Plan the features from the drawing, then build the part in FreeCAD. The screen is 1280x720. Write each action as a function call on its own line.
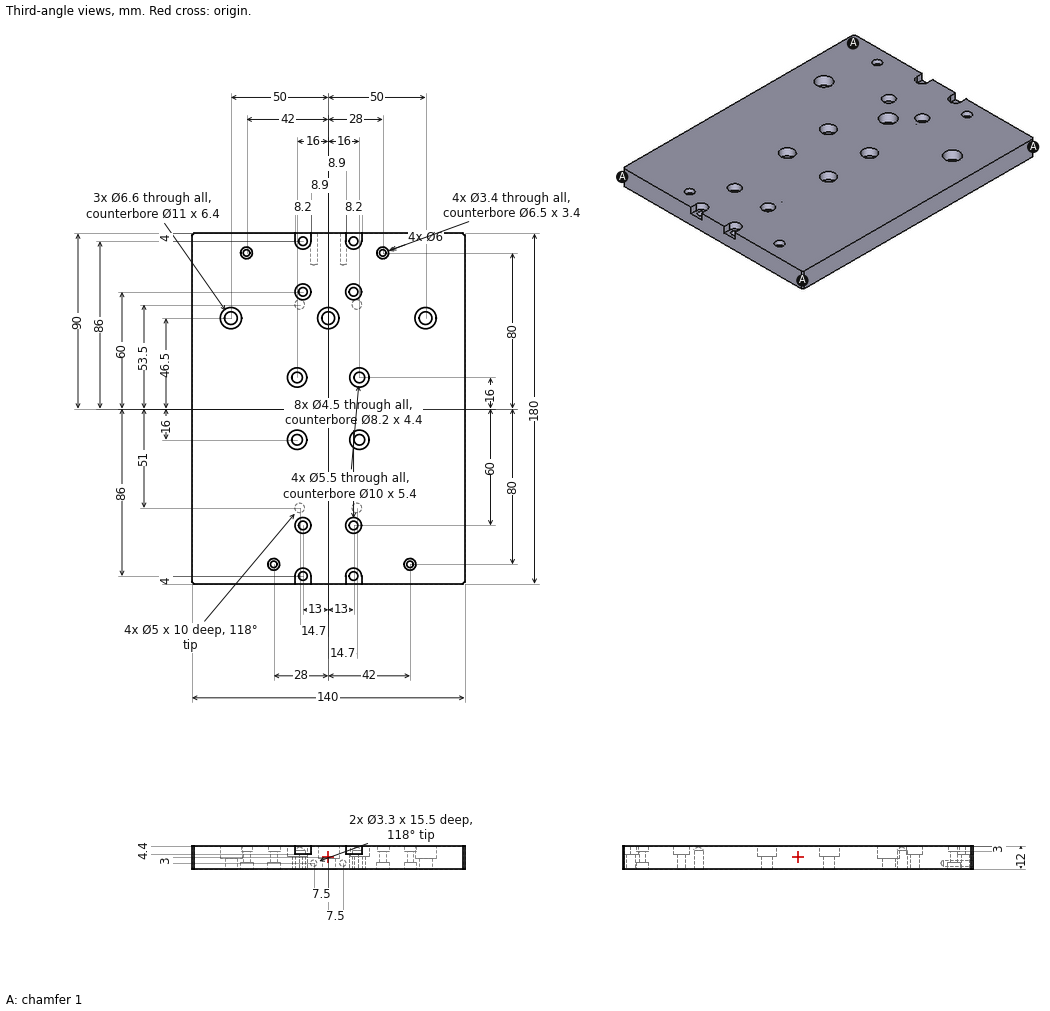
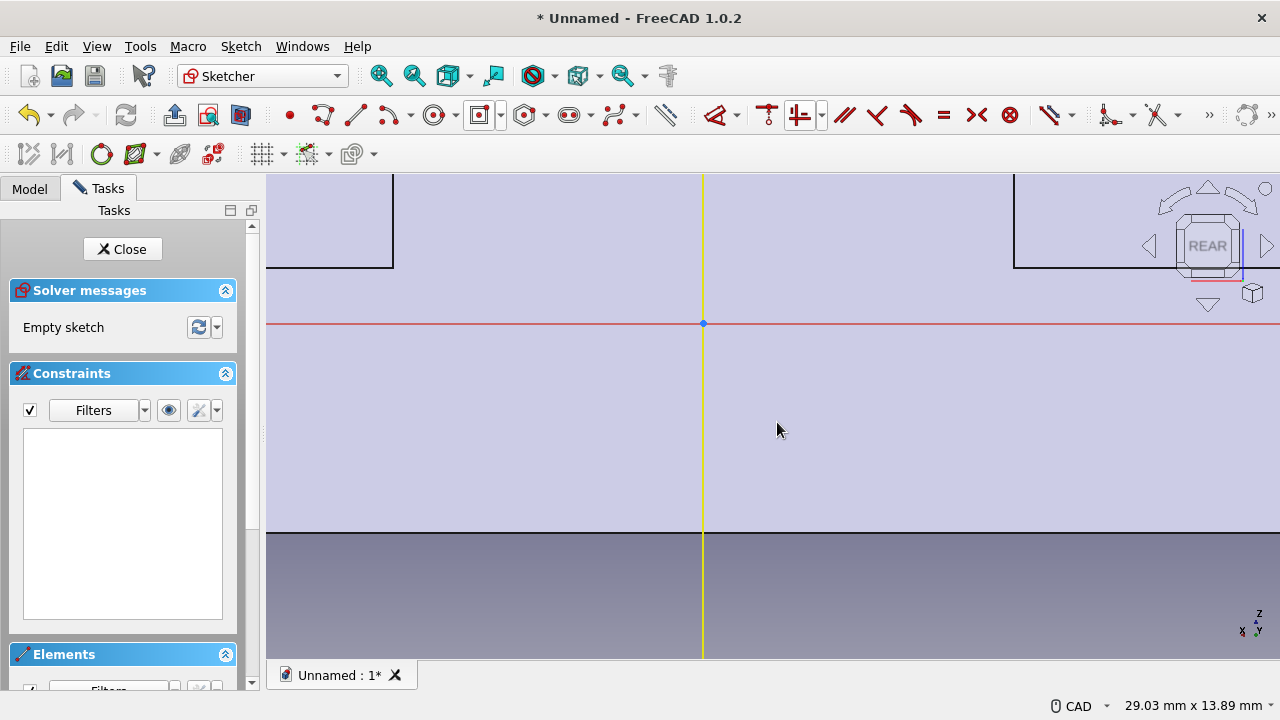
click(434, 116)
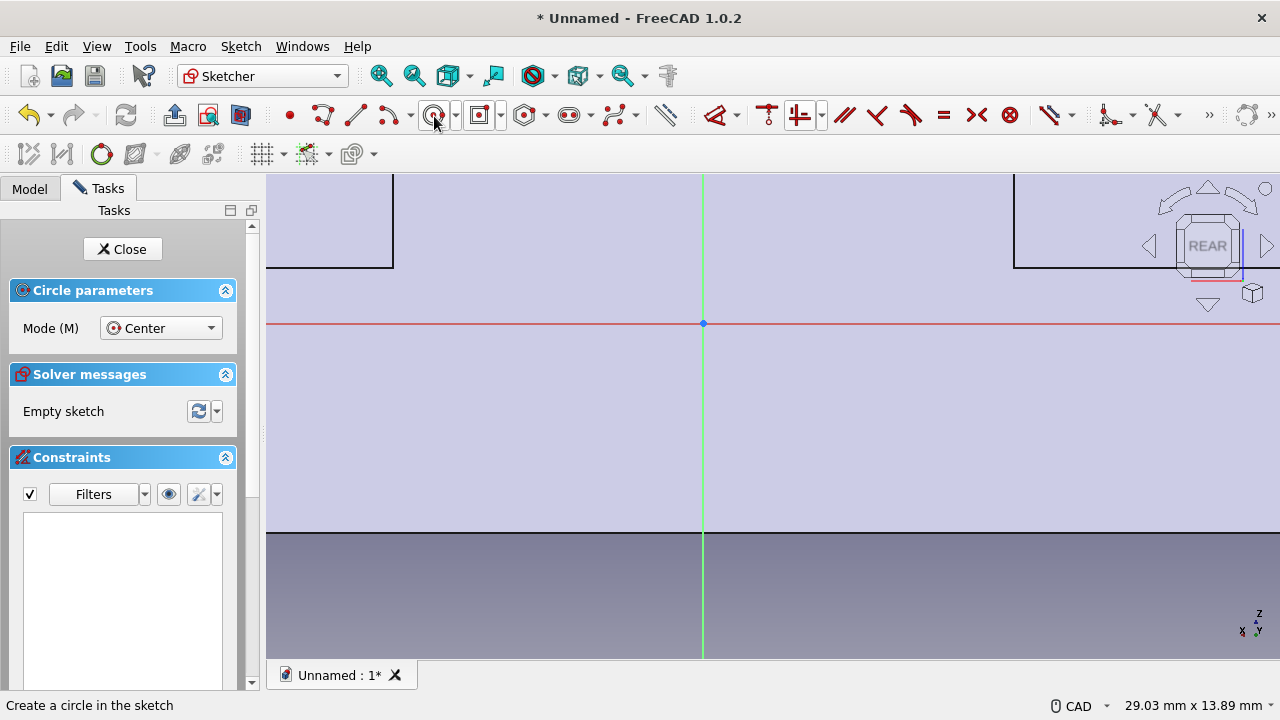
click(965, 428)
click(1006, 388)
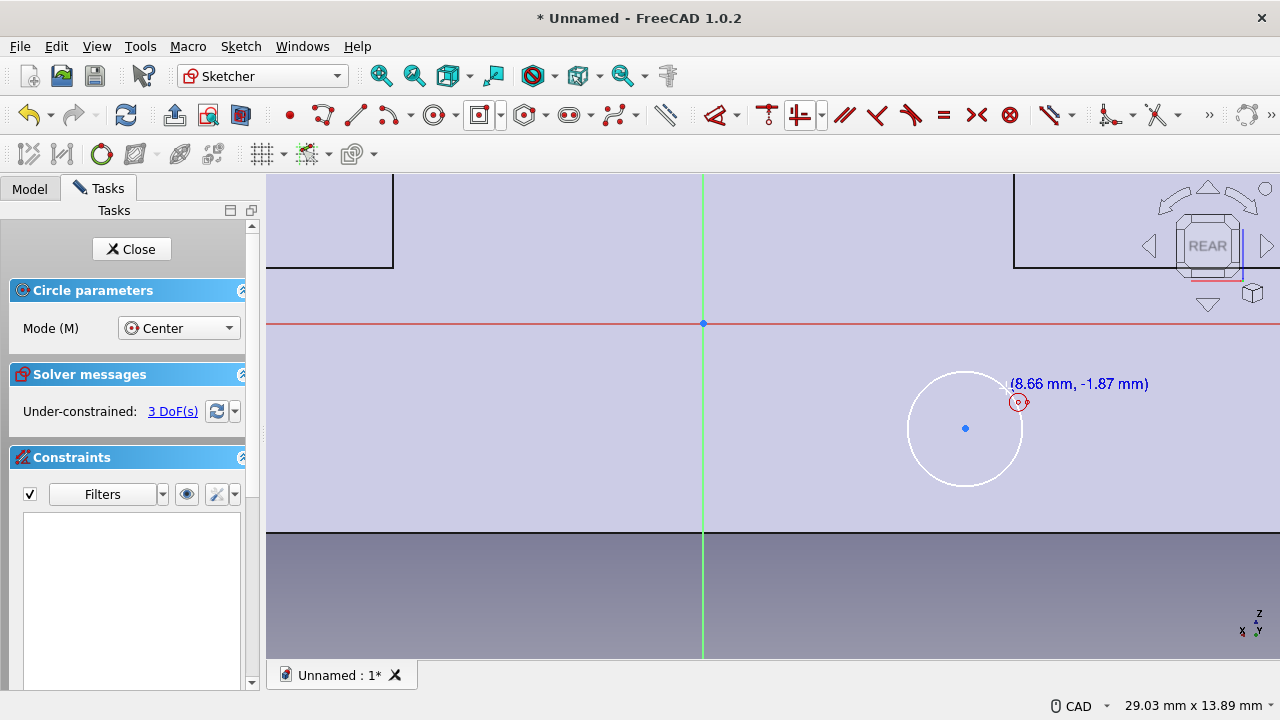
click(441, 428)
click(482, 388)
key(Escape)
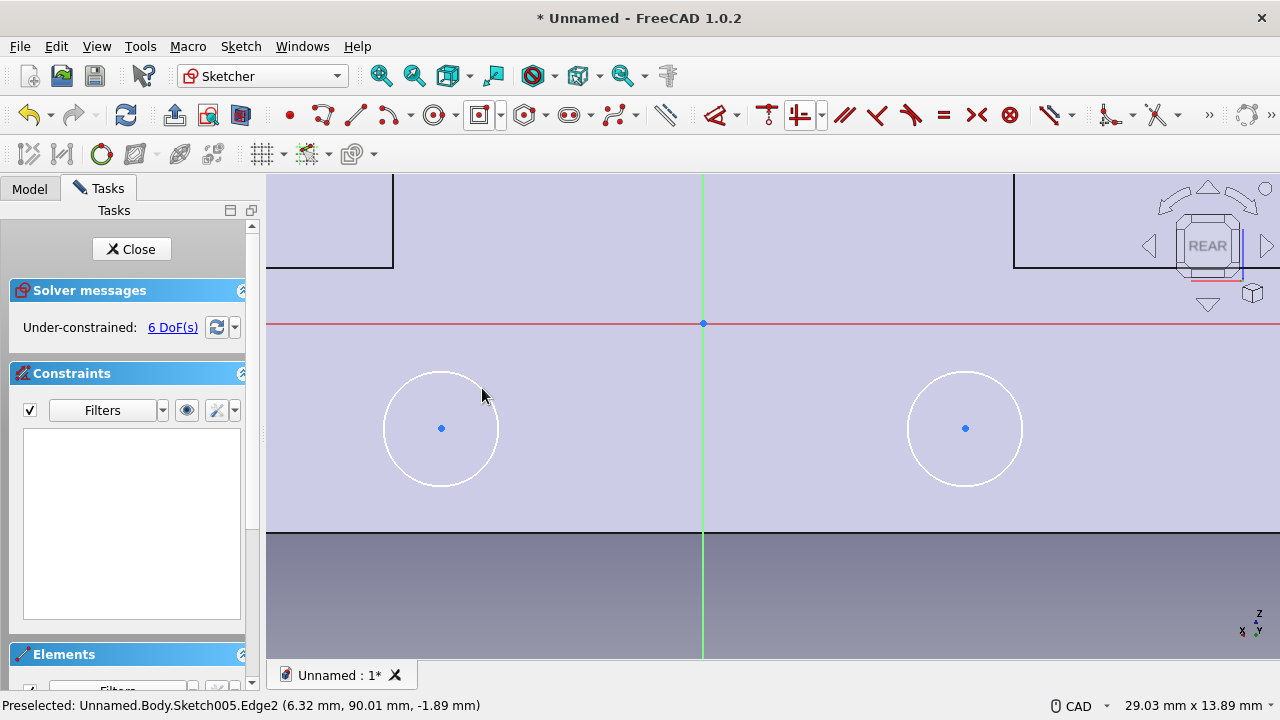
click(1005, 388)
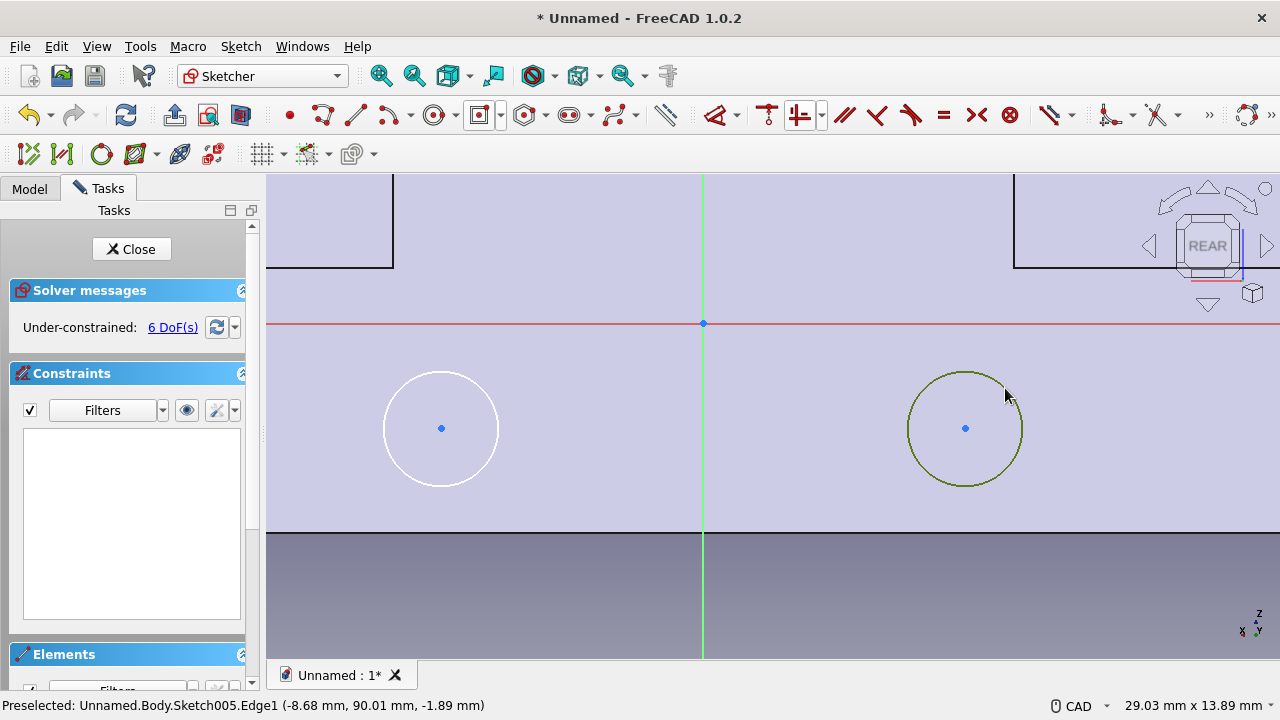
click(481, 388)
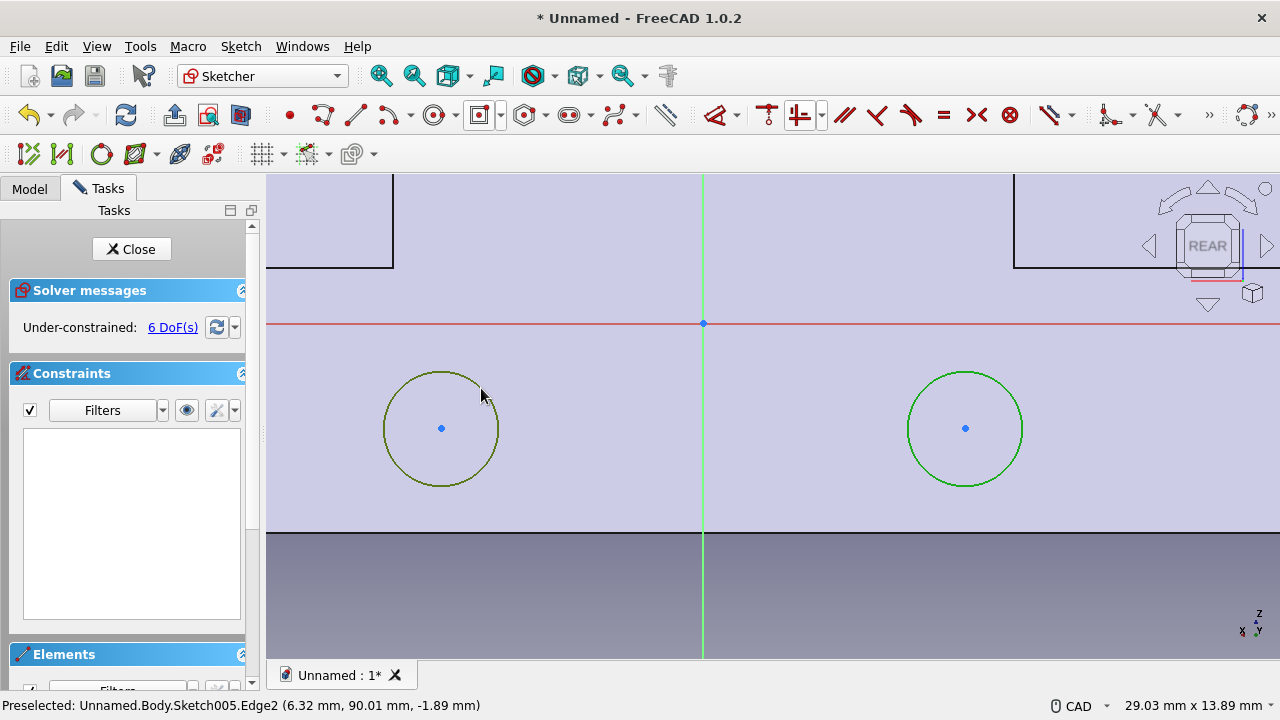
click(944, 116)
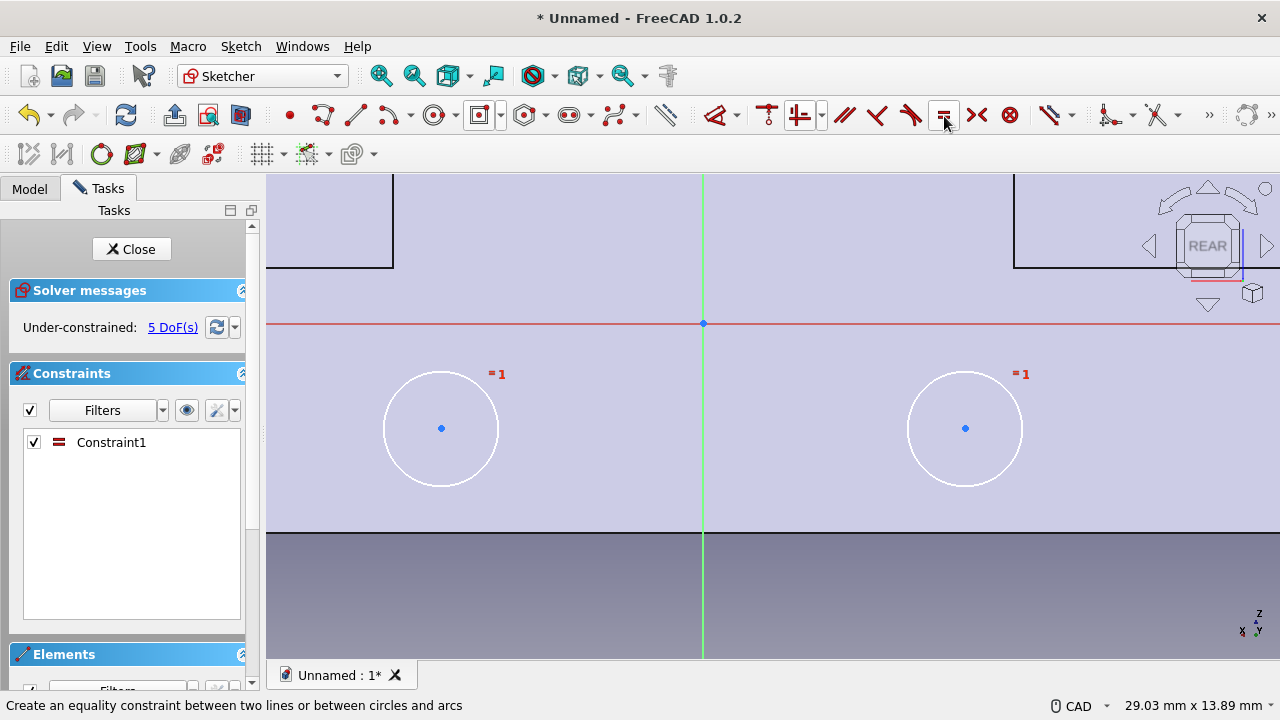
click(714, 116)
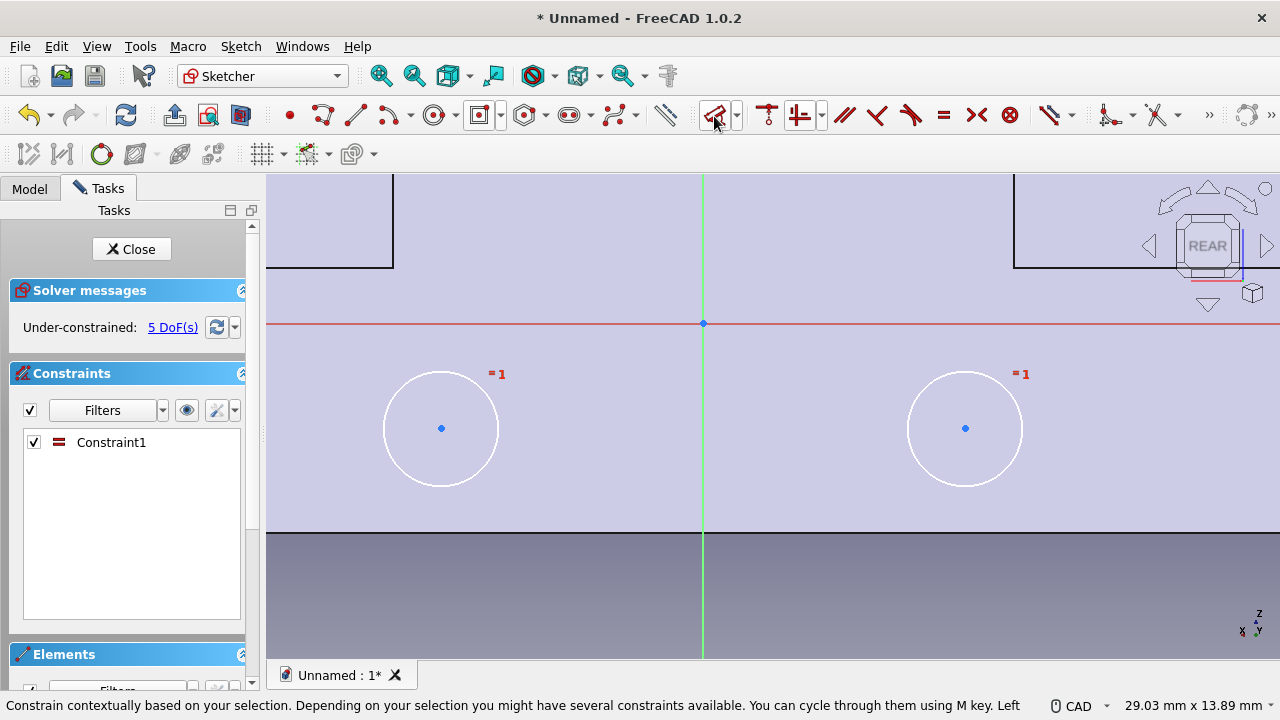
click(1005, 388)
click(1027, 365)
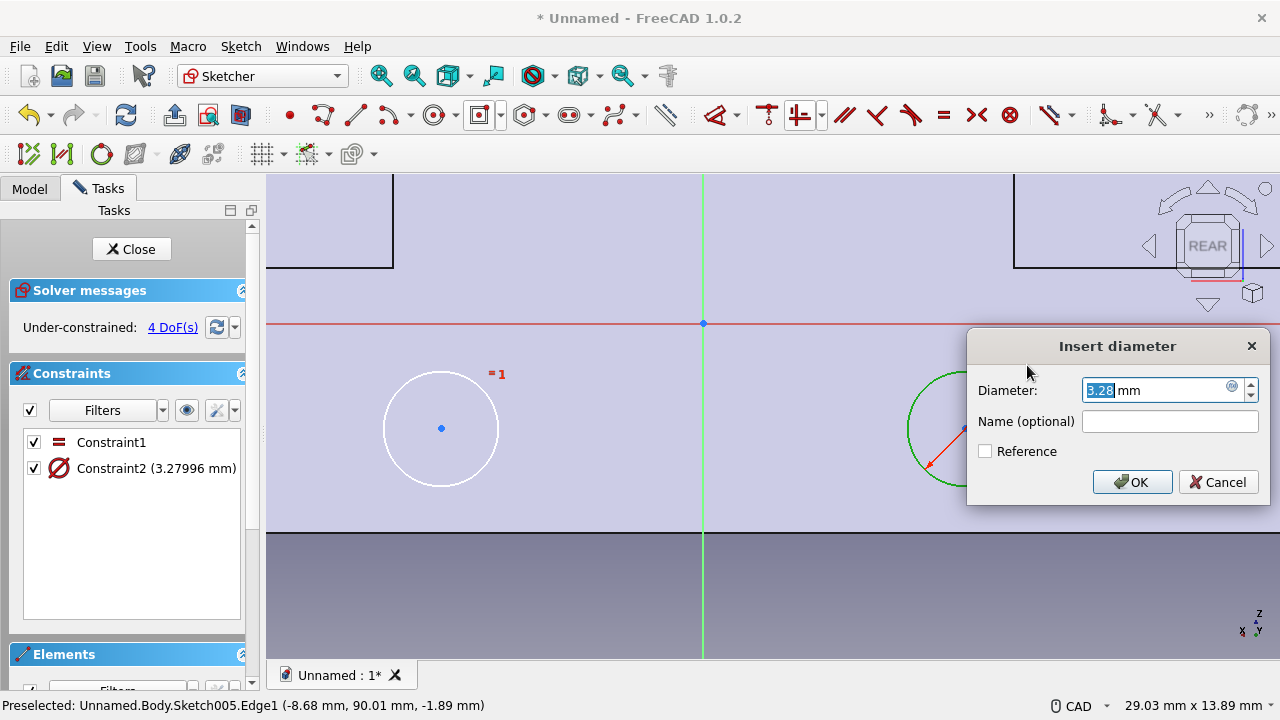
text(3.3)
key(Return)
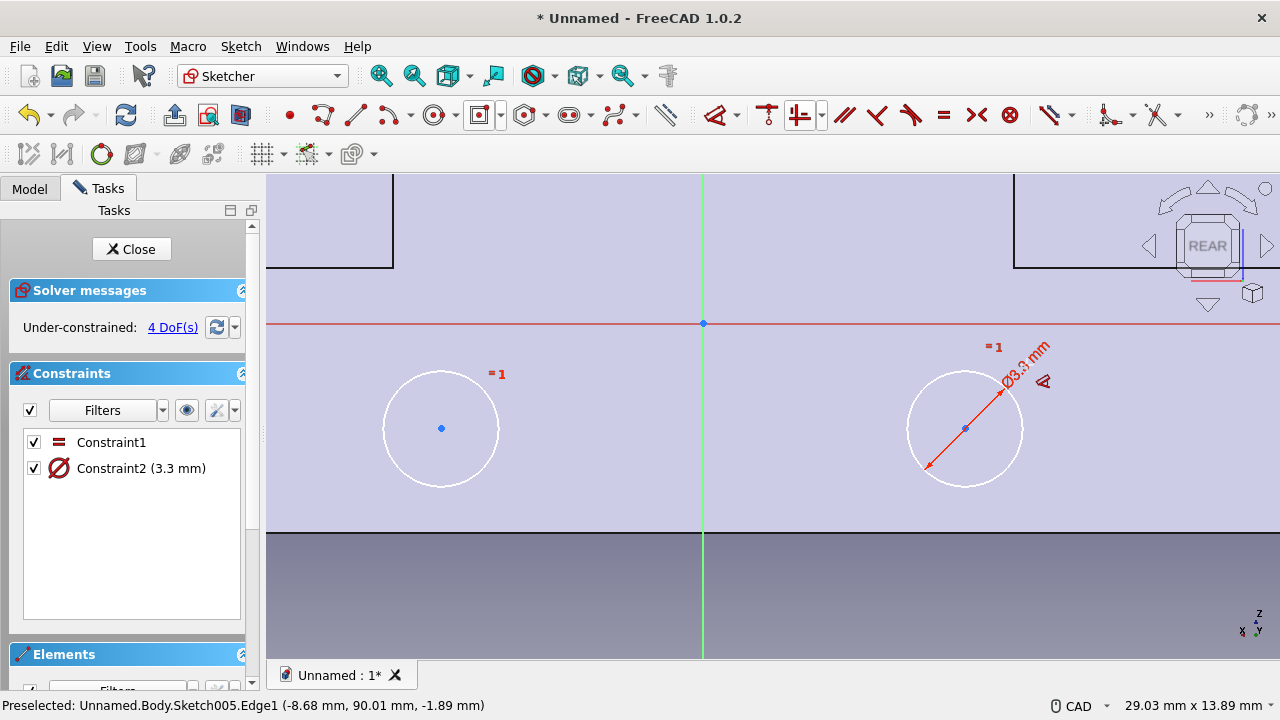
click(965, 429)
click(999, 401)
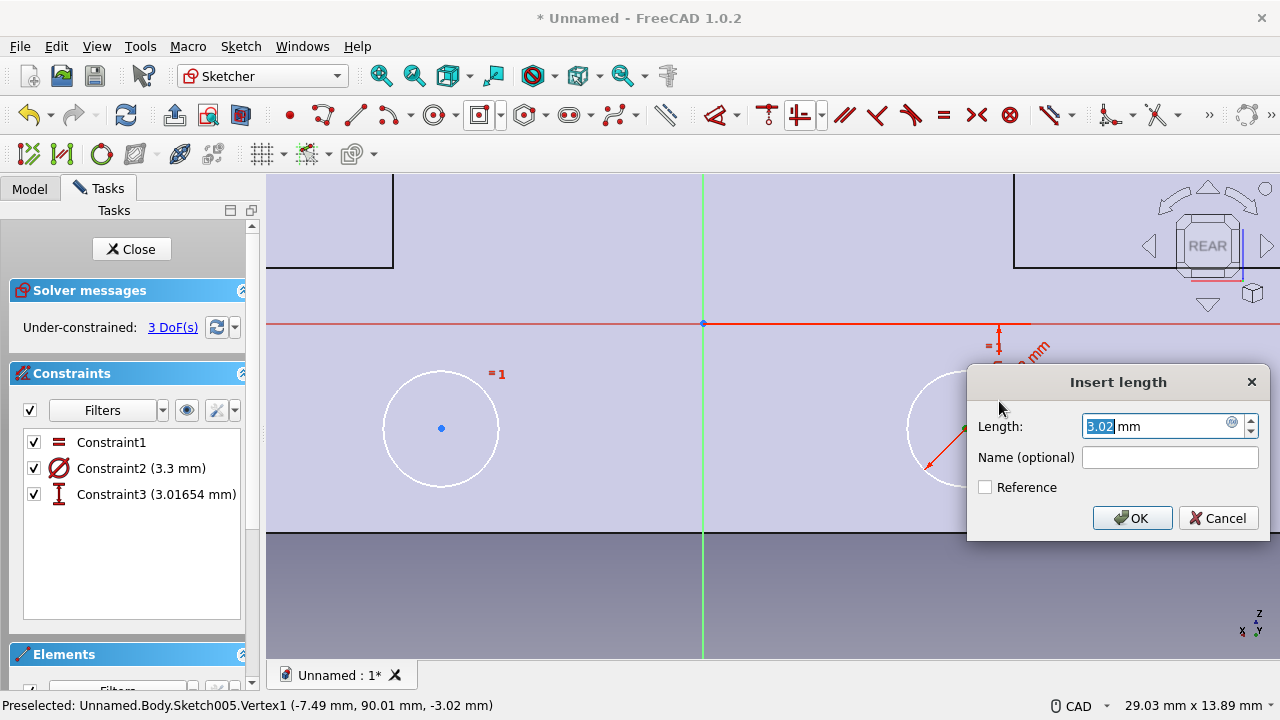
text(3)
key(Return)